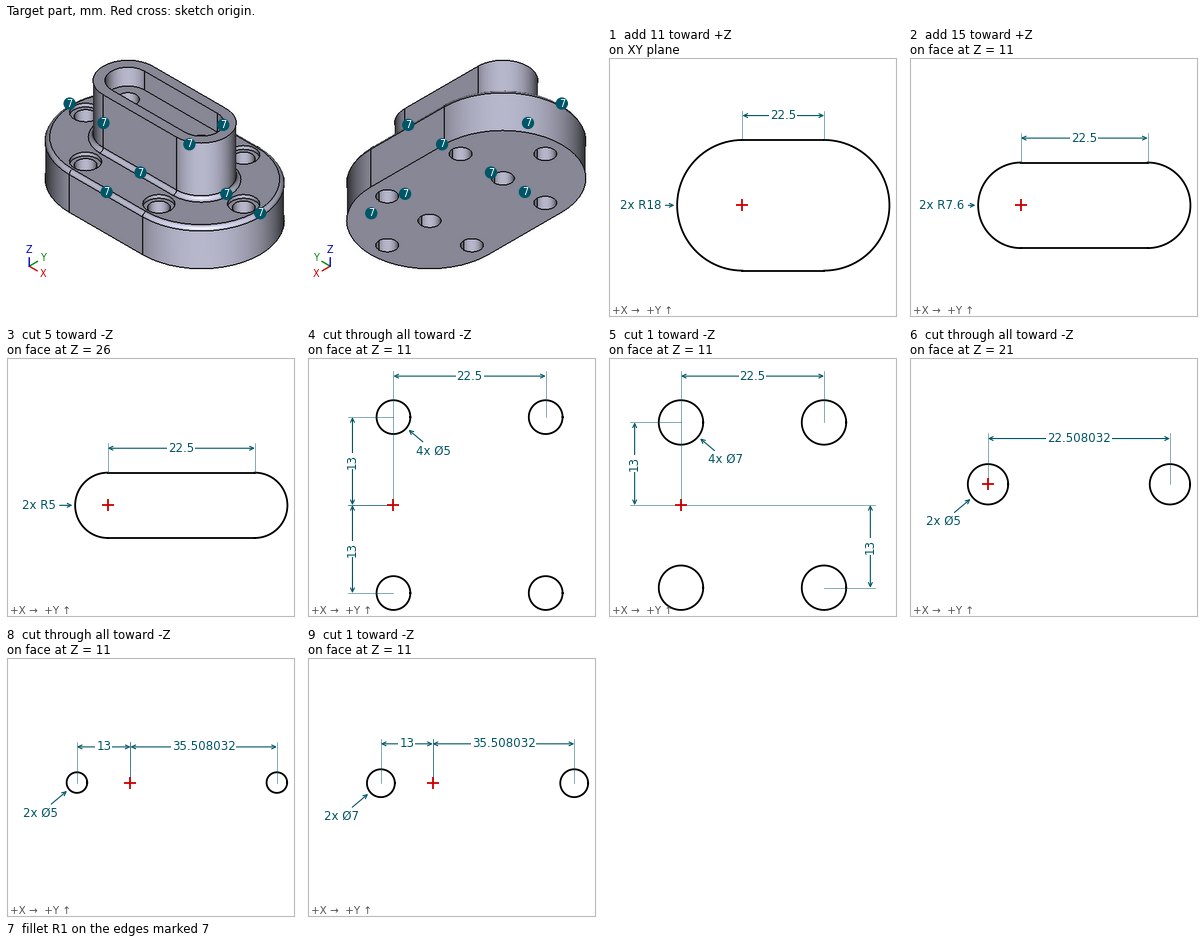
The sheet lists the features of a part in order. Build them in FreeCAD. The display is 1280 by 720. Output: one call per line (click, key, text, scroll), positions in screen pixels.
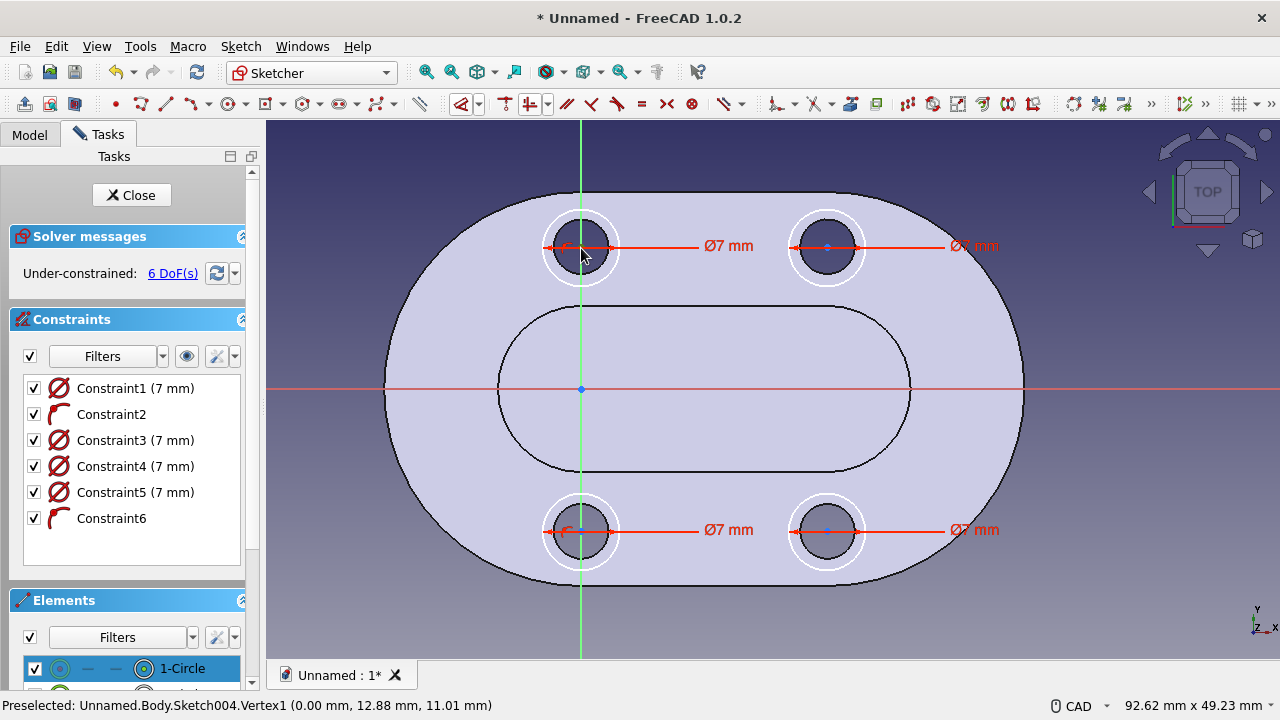
click(827, 248)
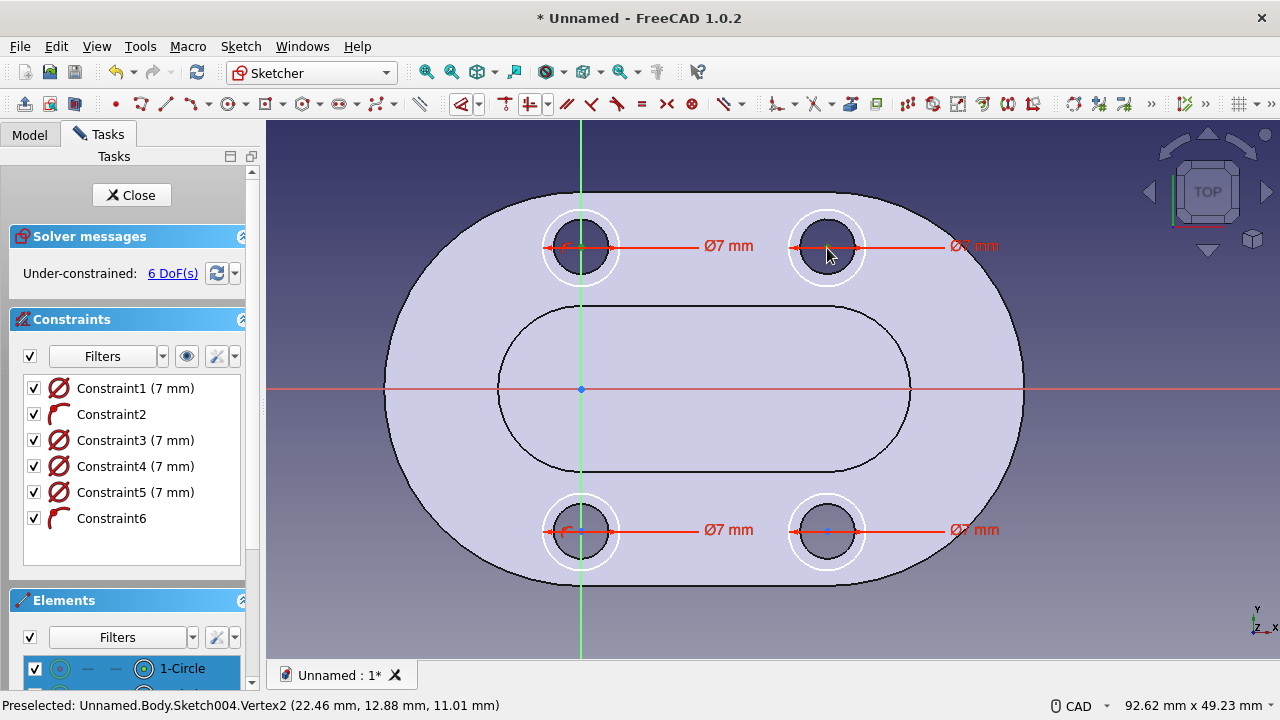
key(h)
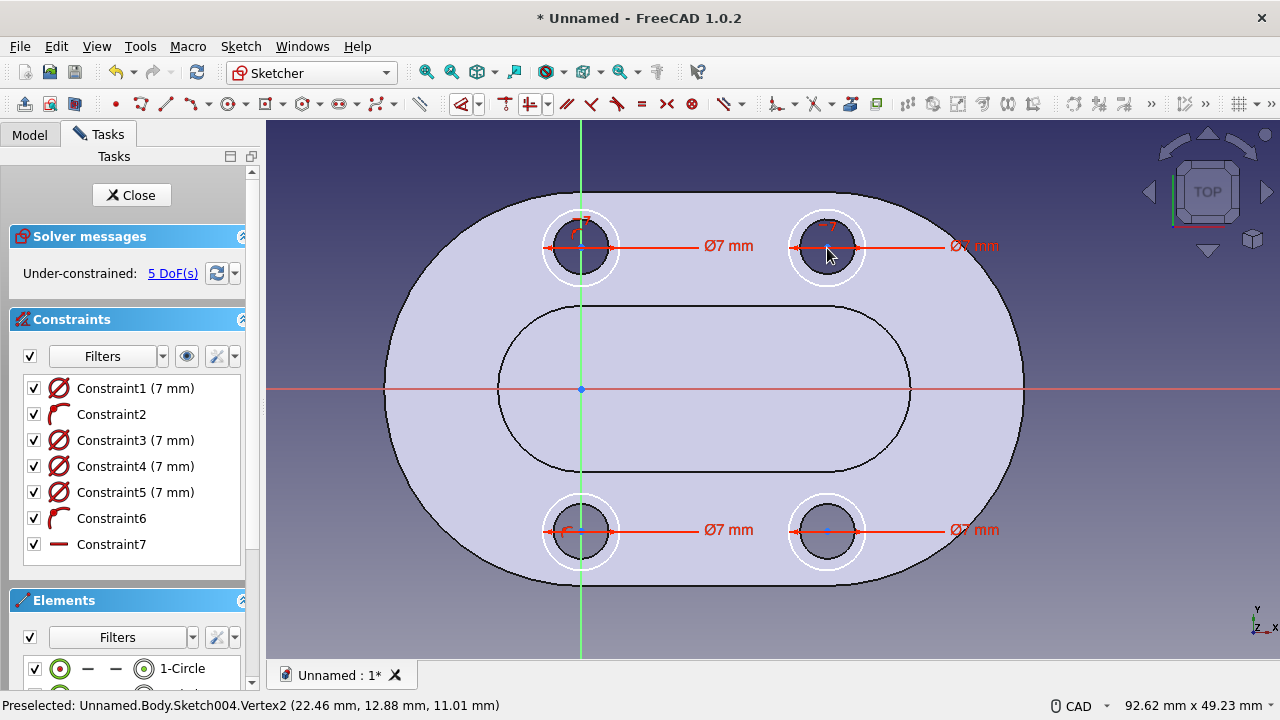
click(827, 248)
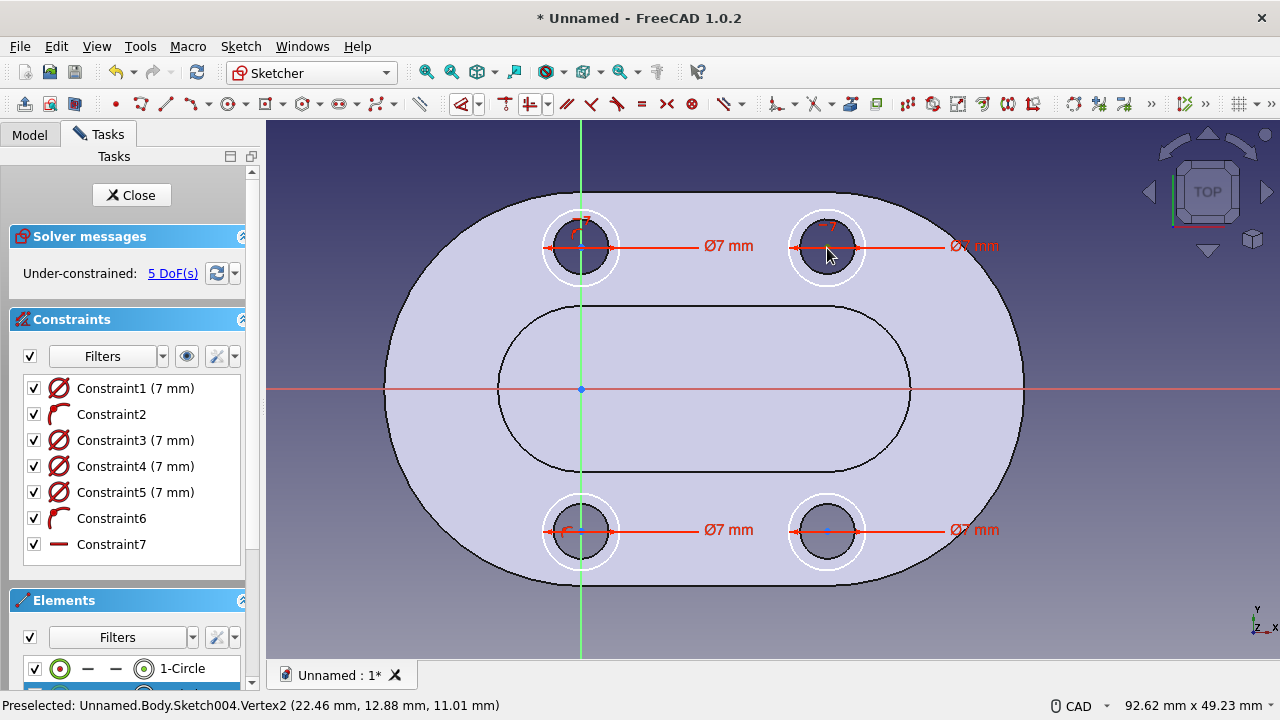
click(827, 532)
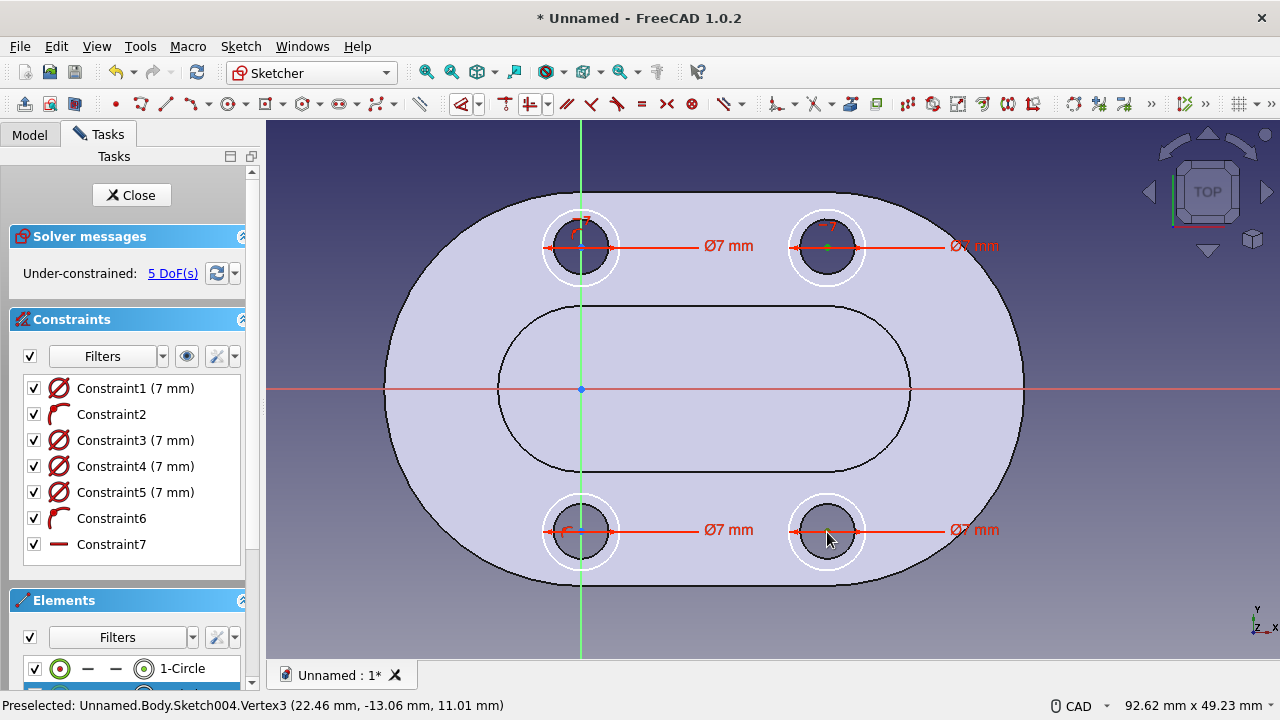
key(v)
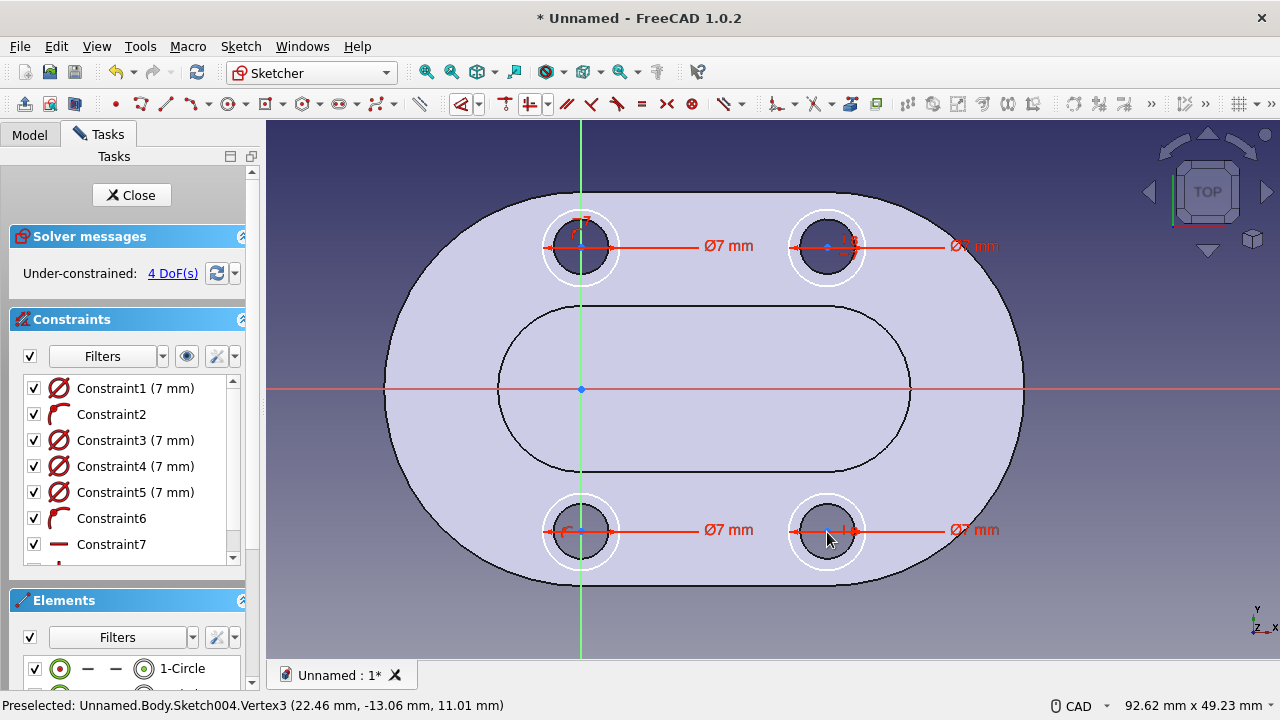
click(827, 532)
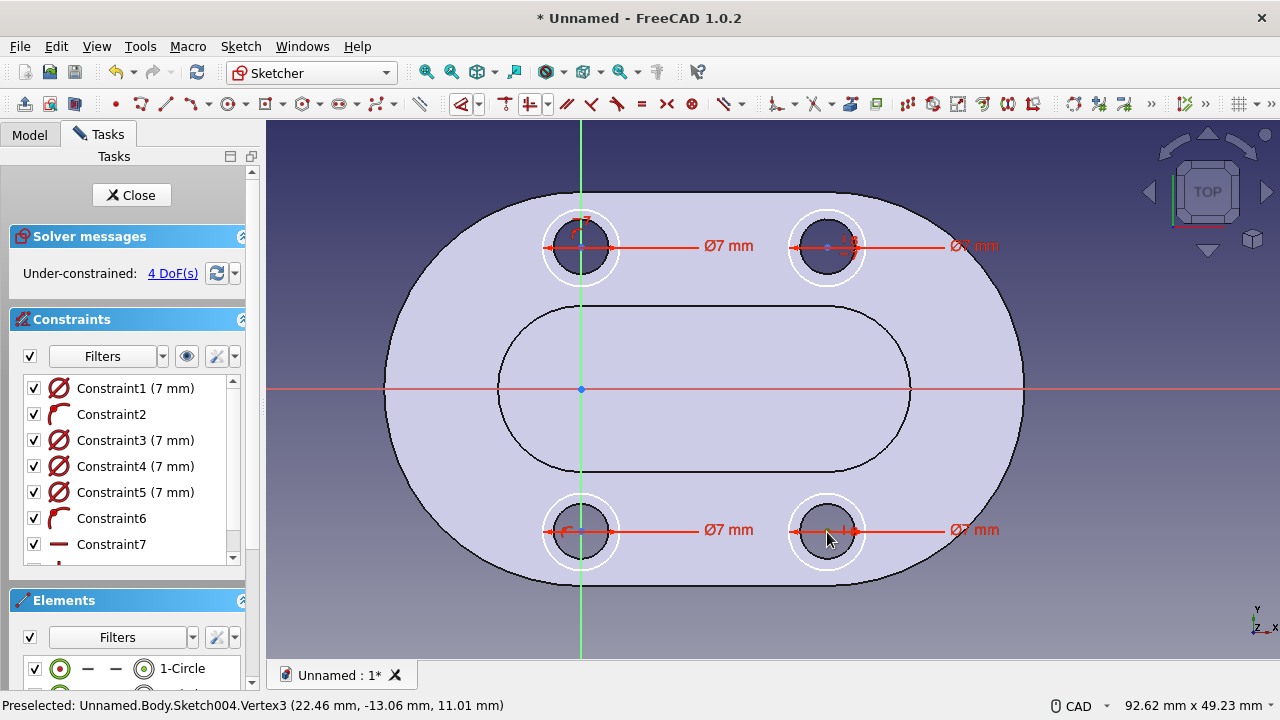
click(581, 532)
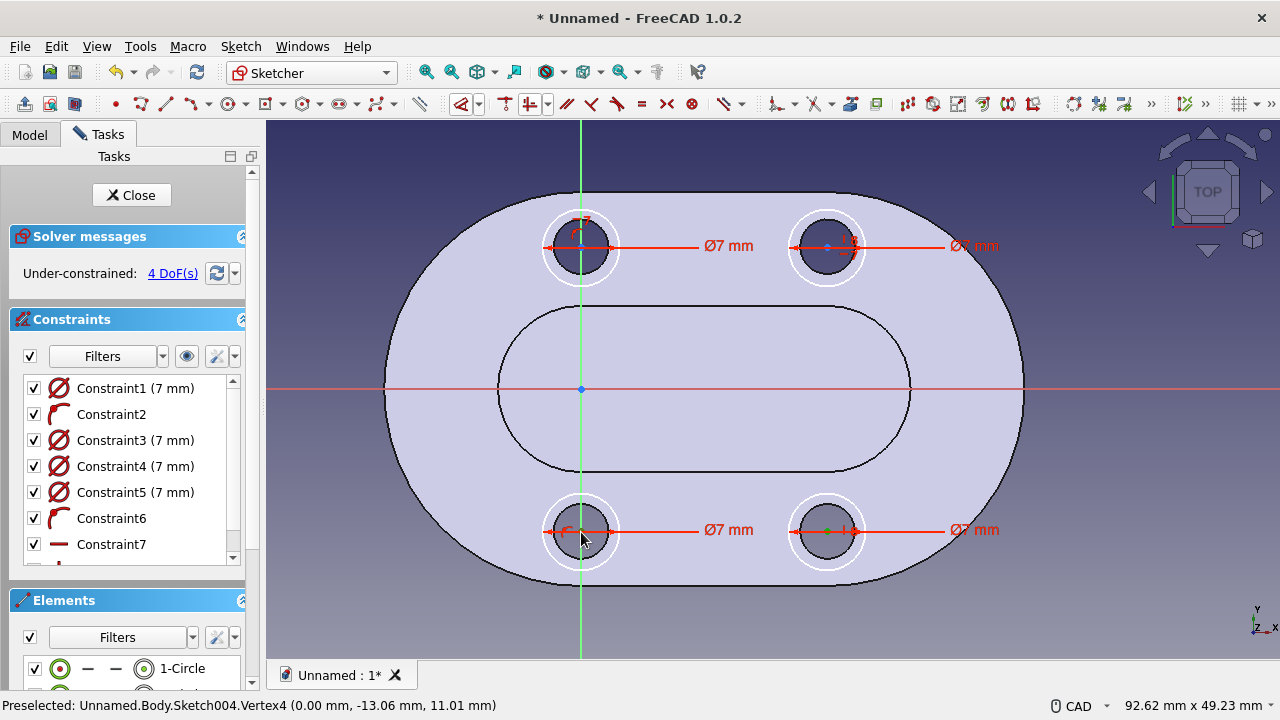
key(h)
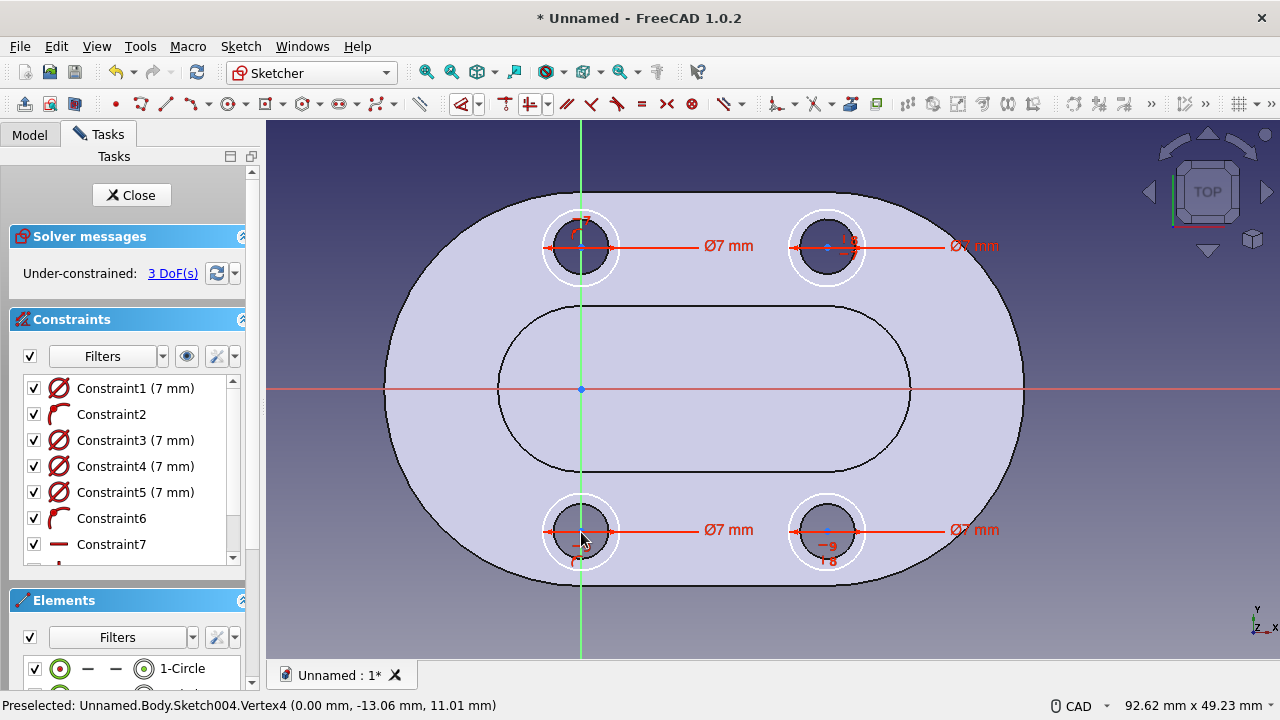
click(581, 248)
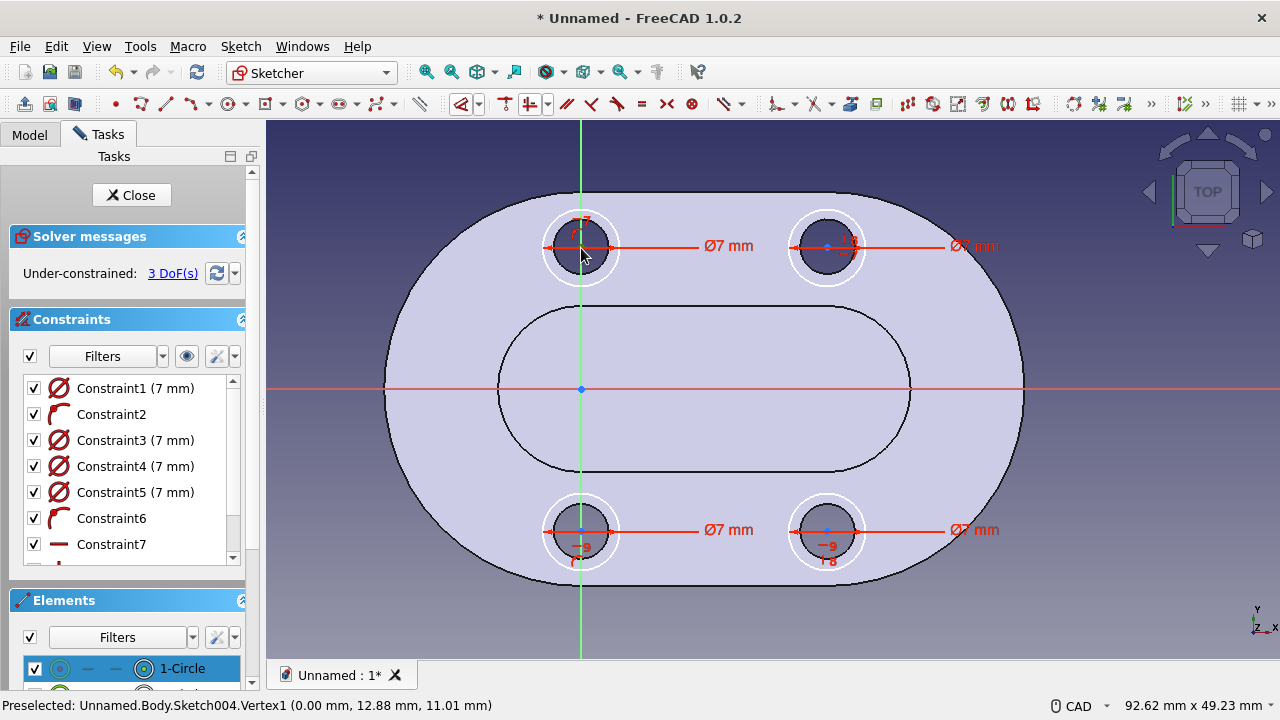
click(478, 104)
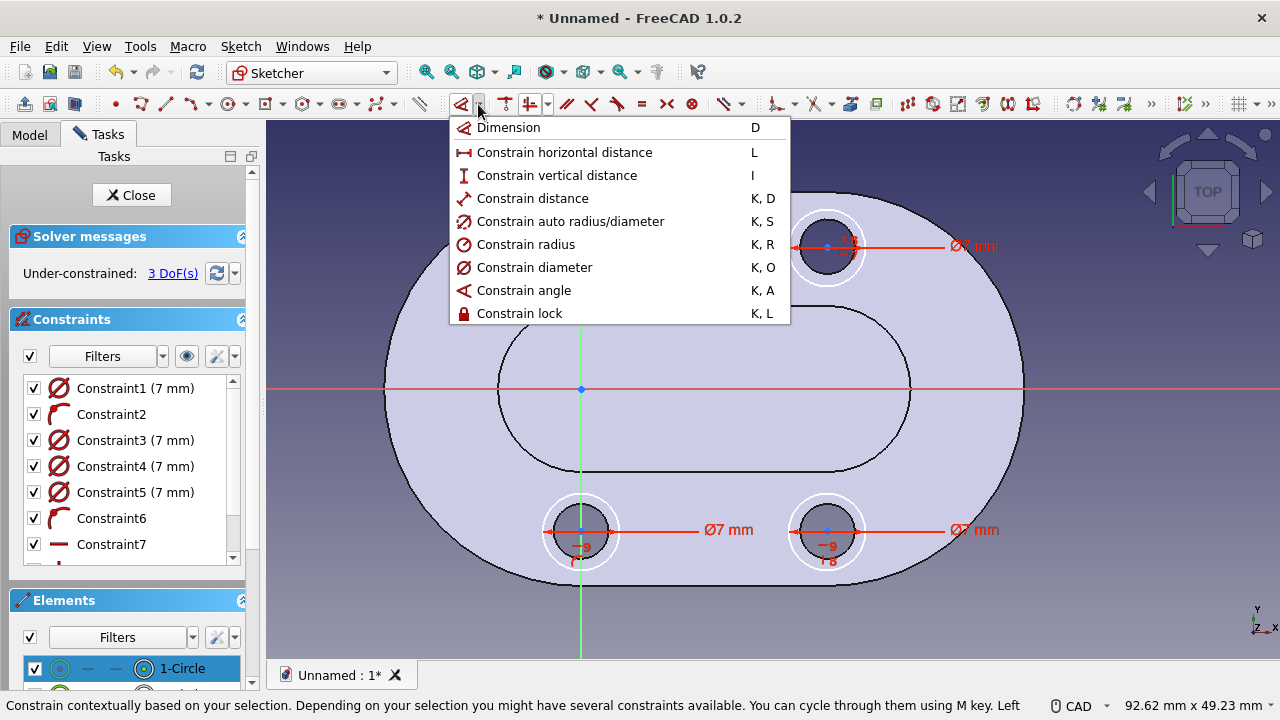
click(620, 176)